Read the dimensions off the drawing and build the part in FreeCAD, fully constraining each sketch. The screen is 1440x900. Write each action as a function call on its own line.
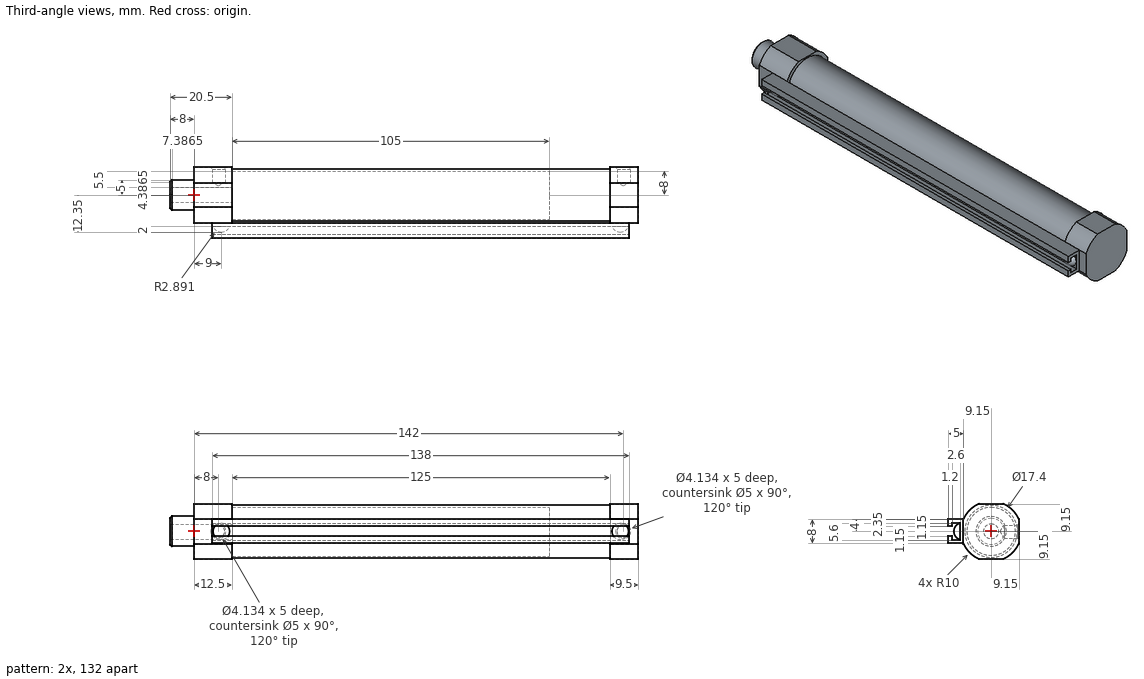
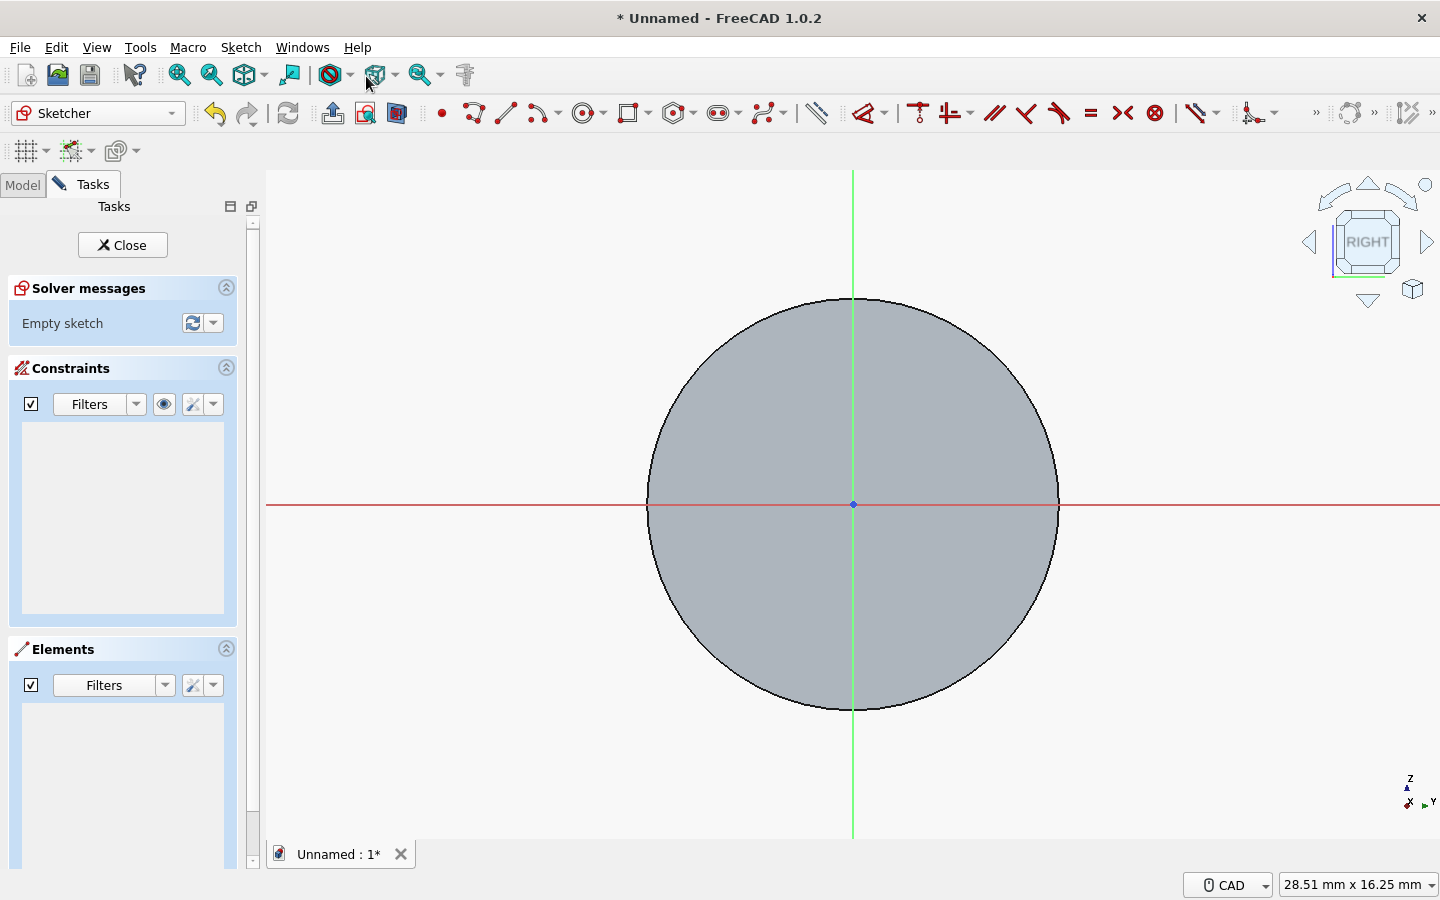
scroll(701, 504, down, 3)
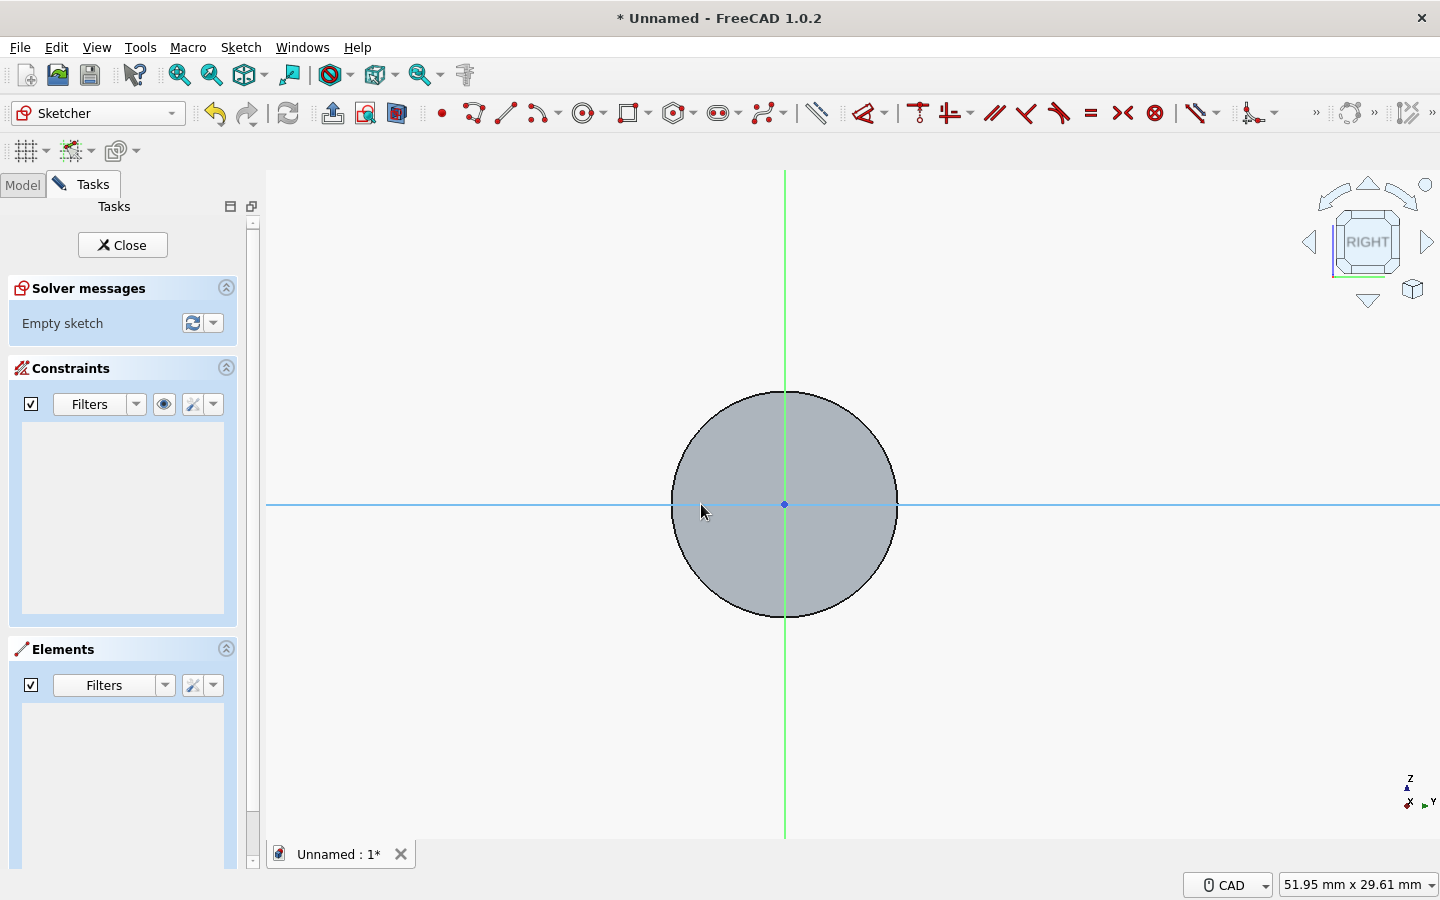
click(506, 114)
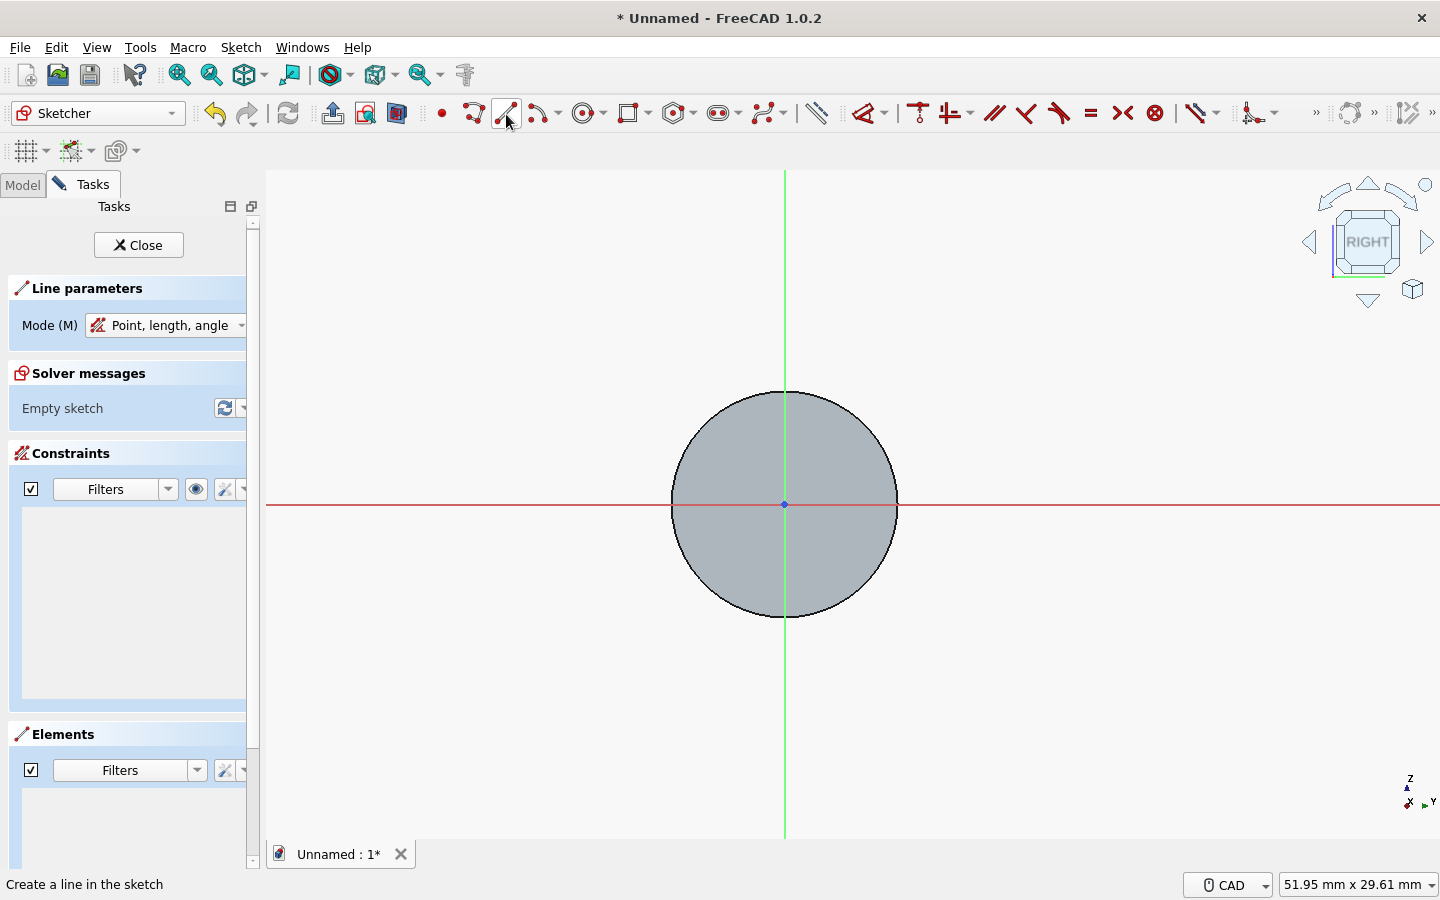
click(578, 413)
click(578, 596)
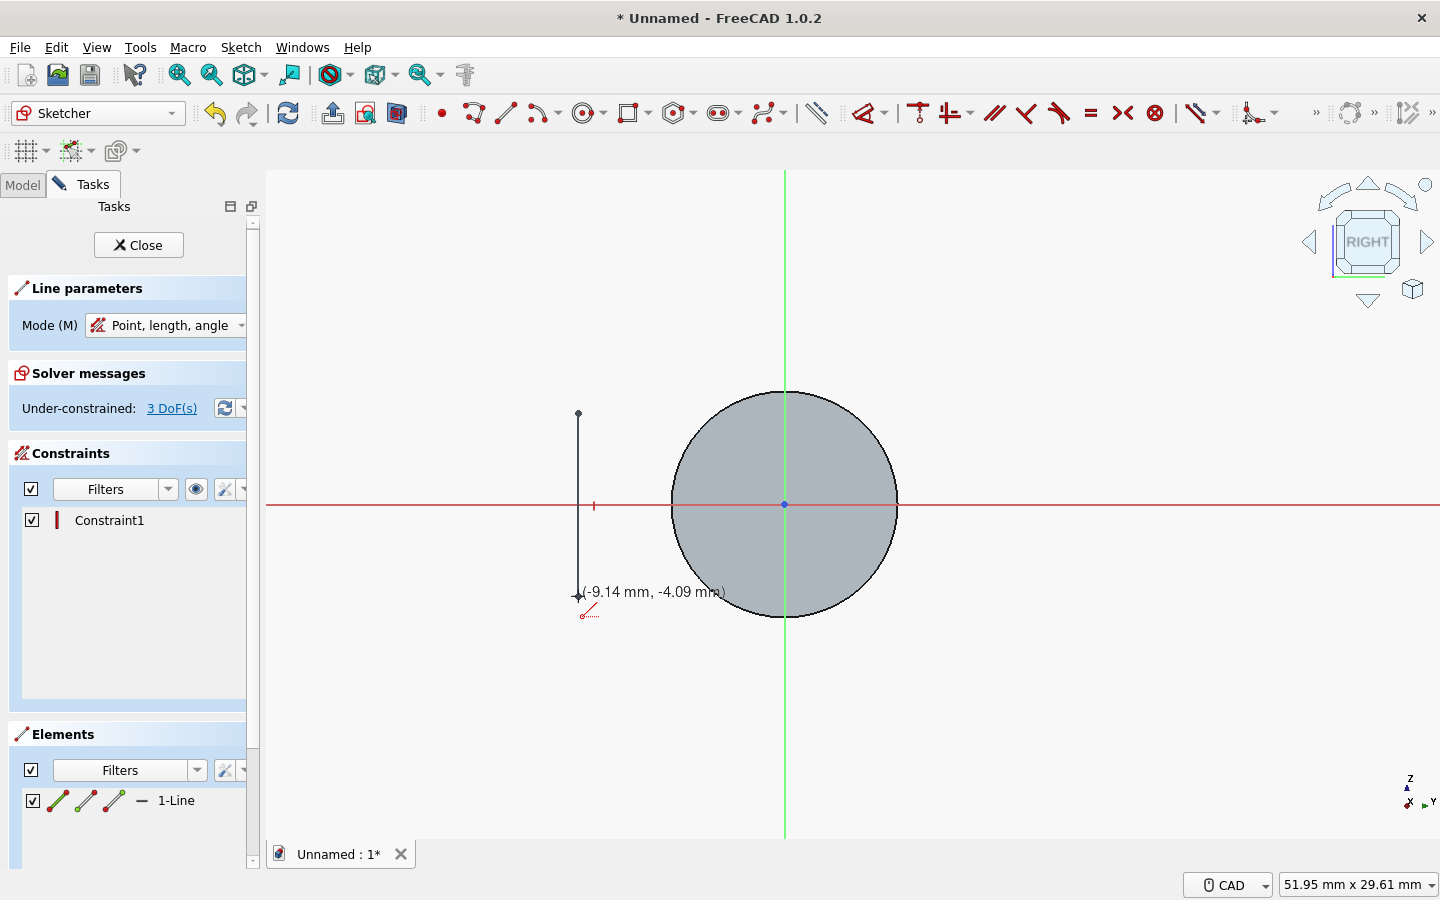
click(693, 711)
click(876, 711)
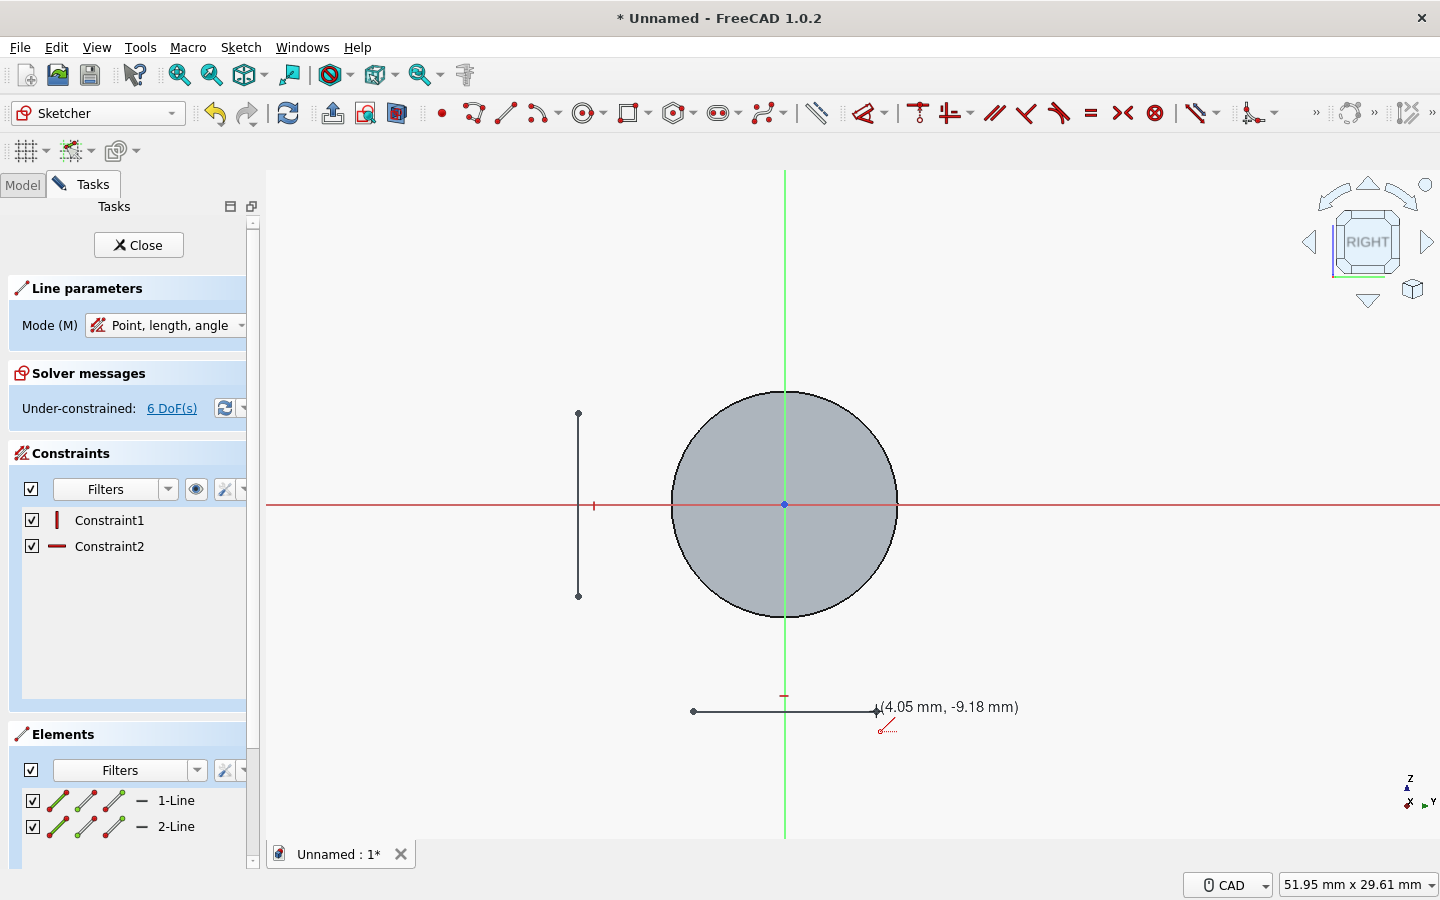
click(991, 596)
click(991, 413)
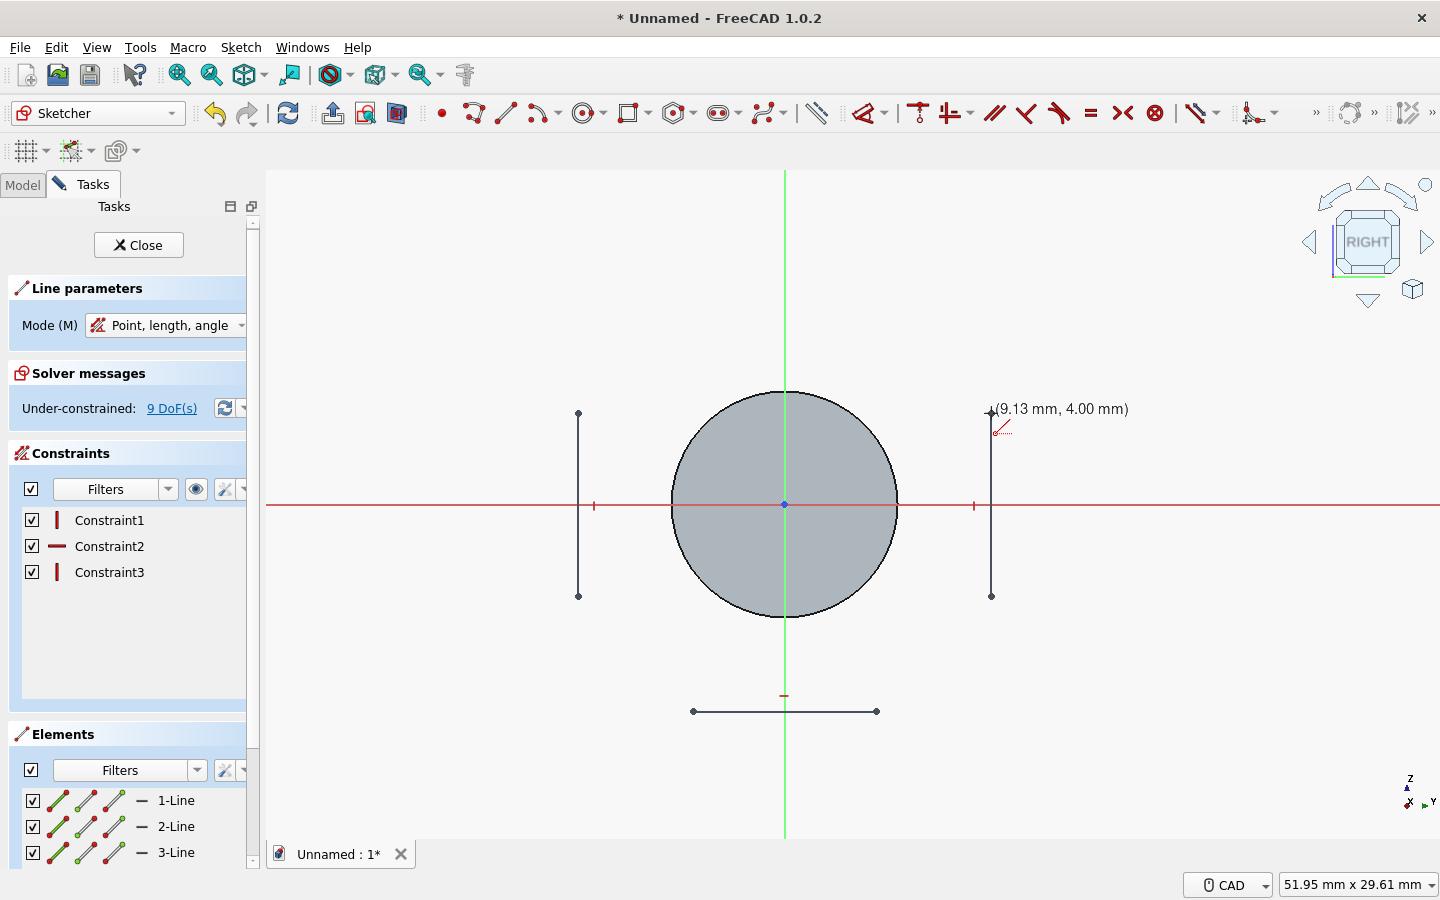
click(876, 298)
click(693, 298)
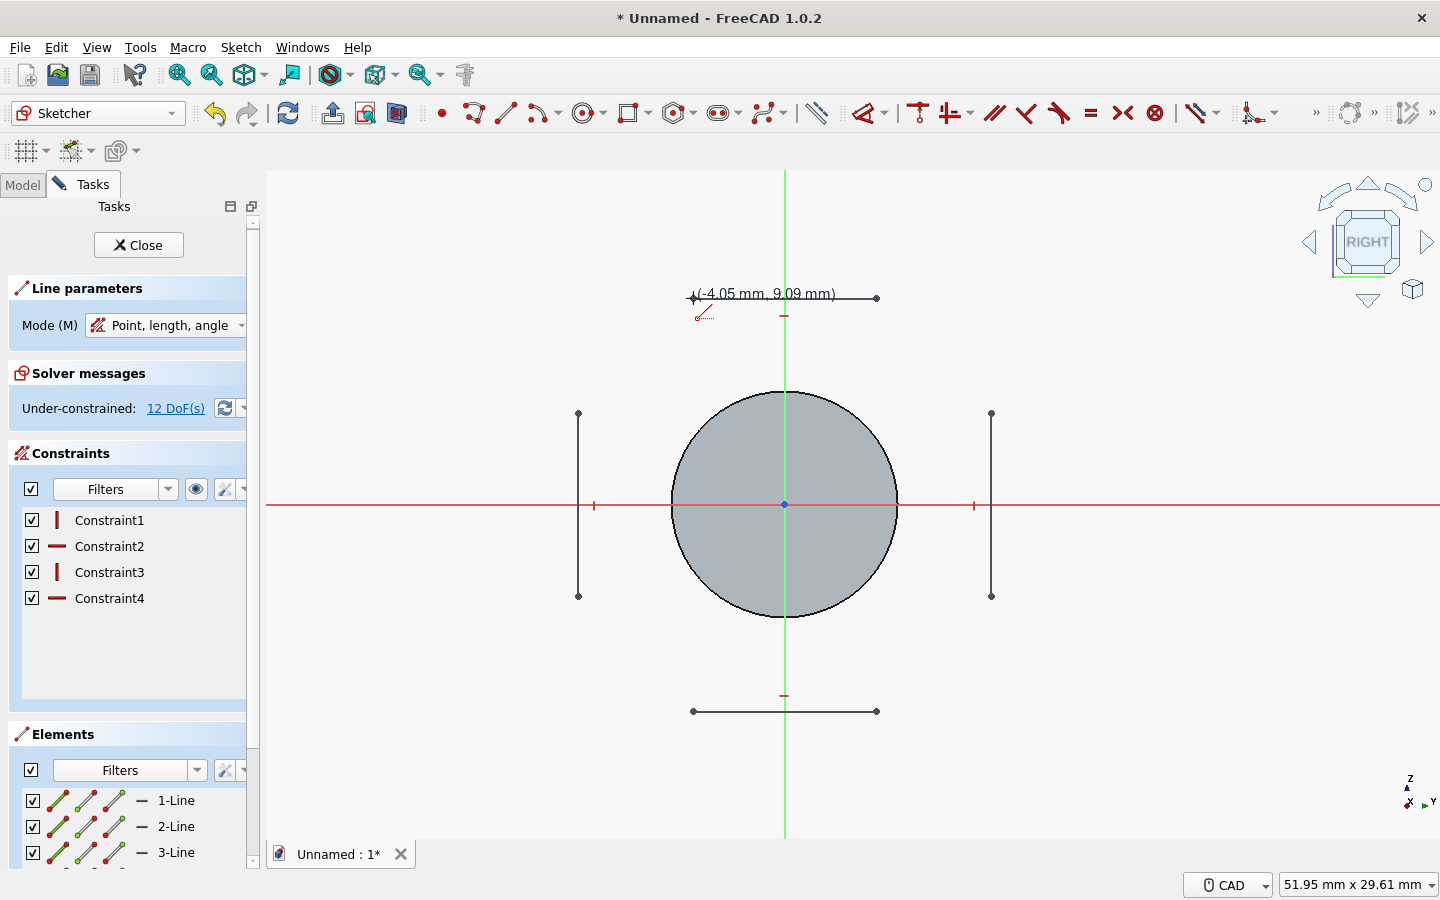
key(g)
key(3)
key(a)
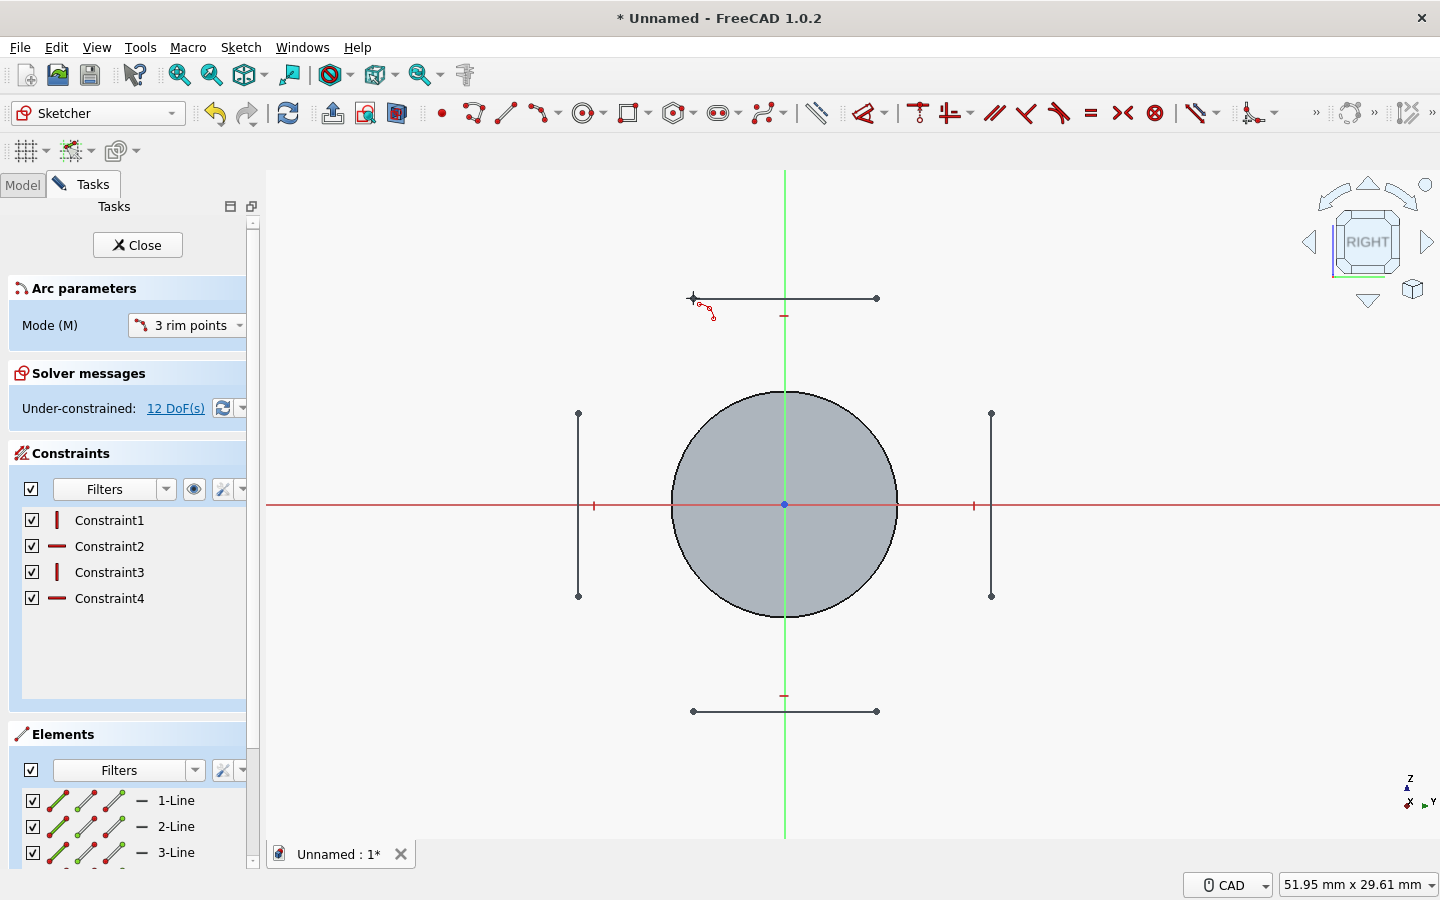
click(578, 597)
click(693, 712)
click(625, 664)